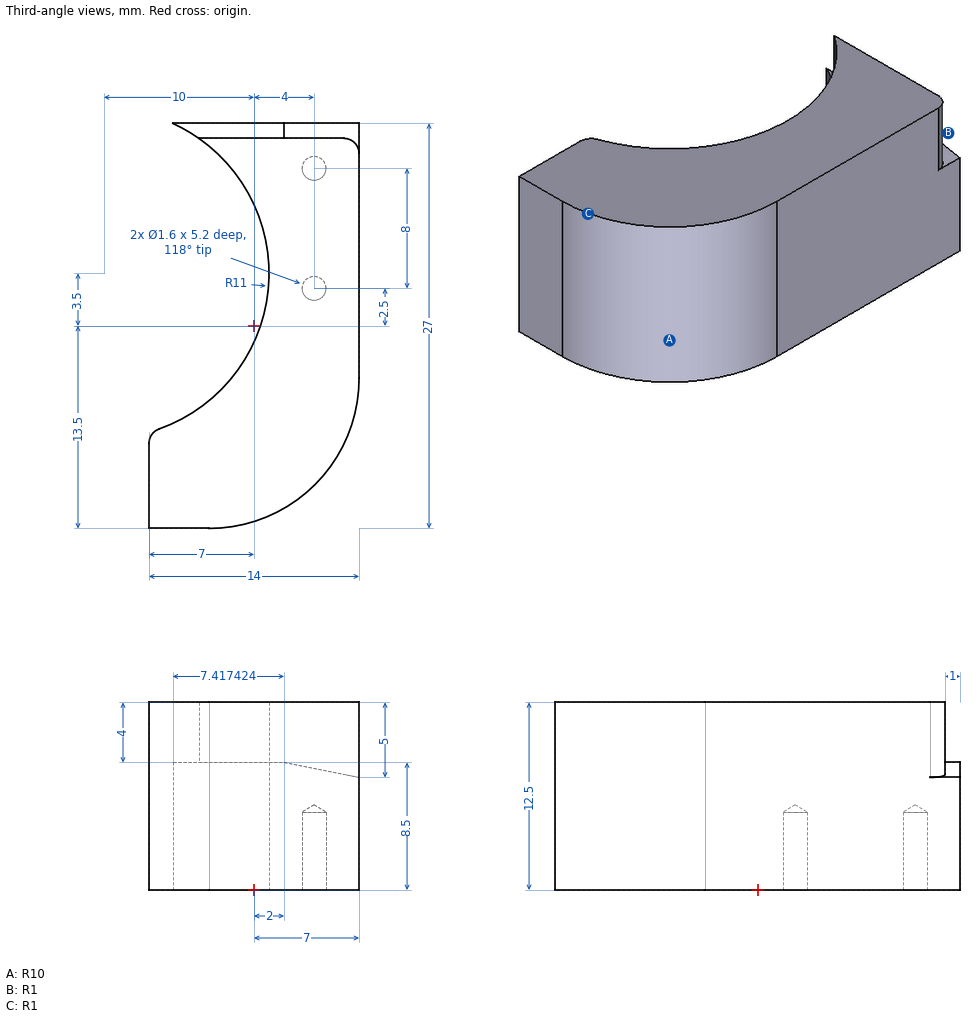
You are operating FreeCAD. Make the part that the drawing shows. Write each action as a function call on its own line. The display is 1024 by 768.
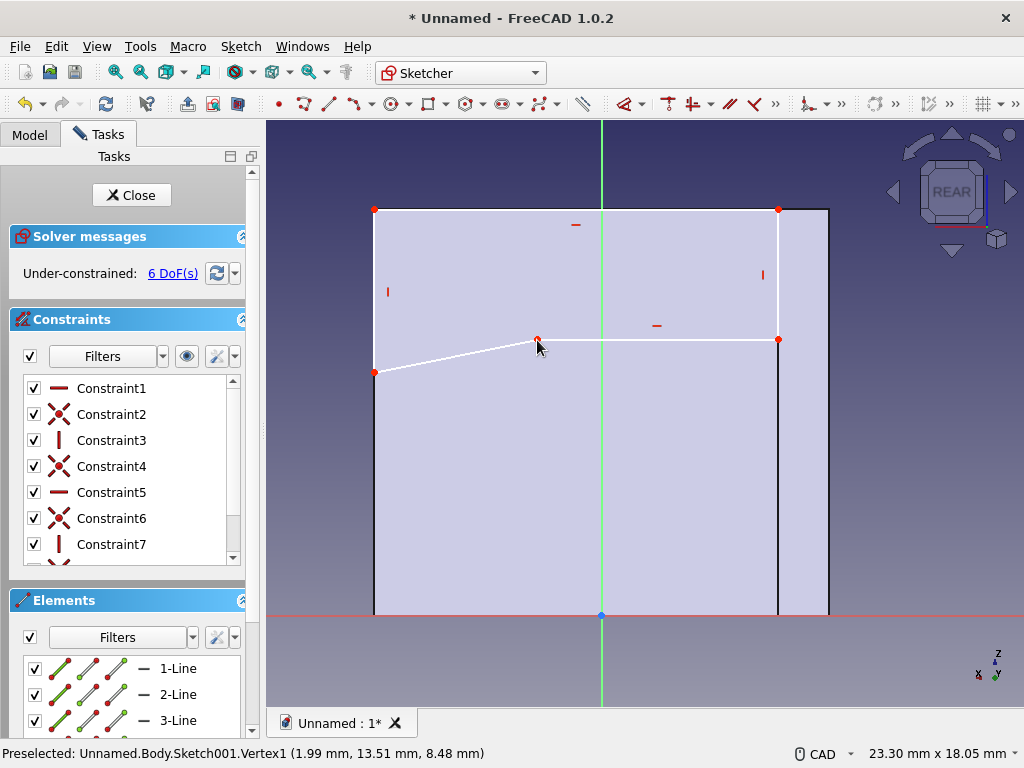
click(624, 104)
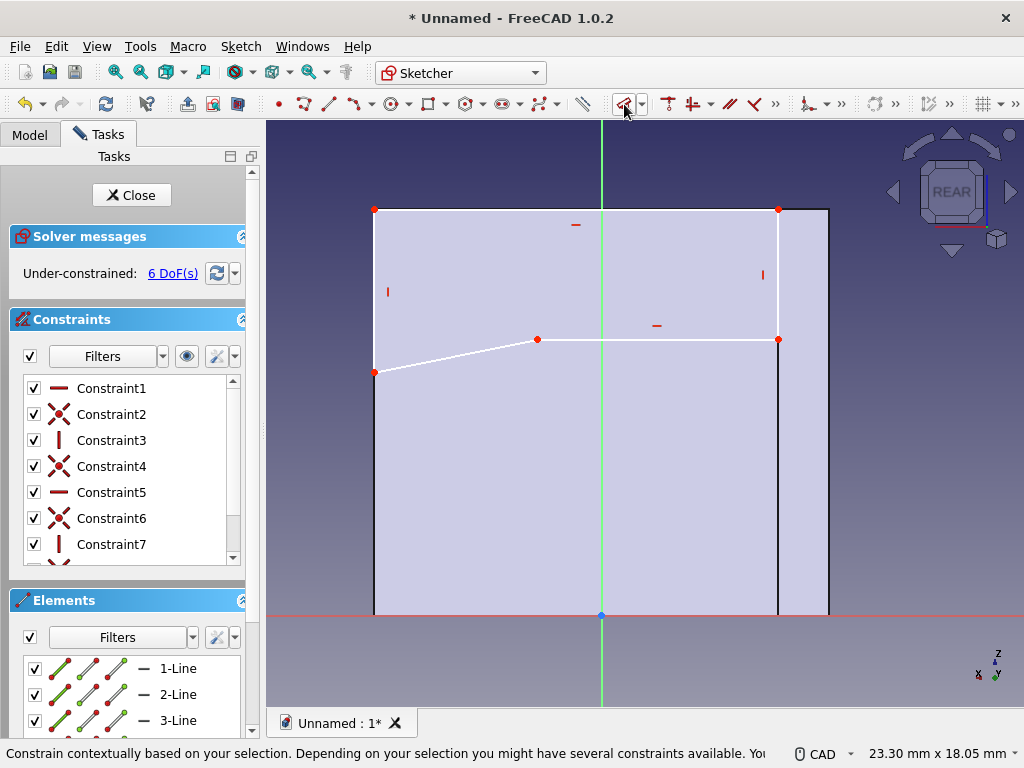
click(778, 301)
click(812, 275)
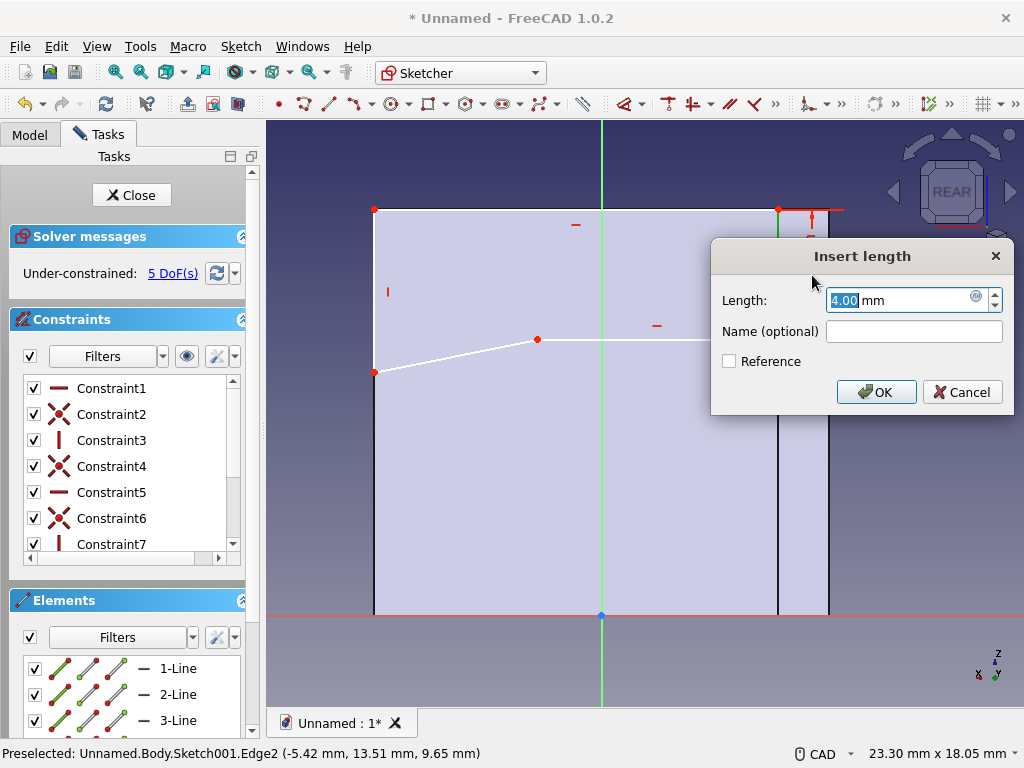
text(4)
key(Return)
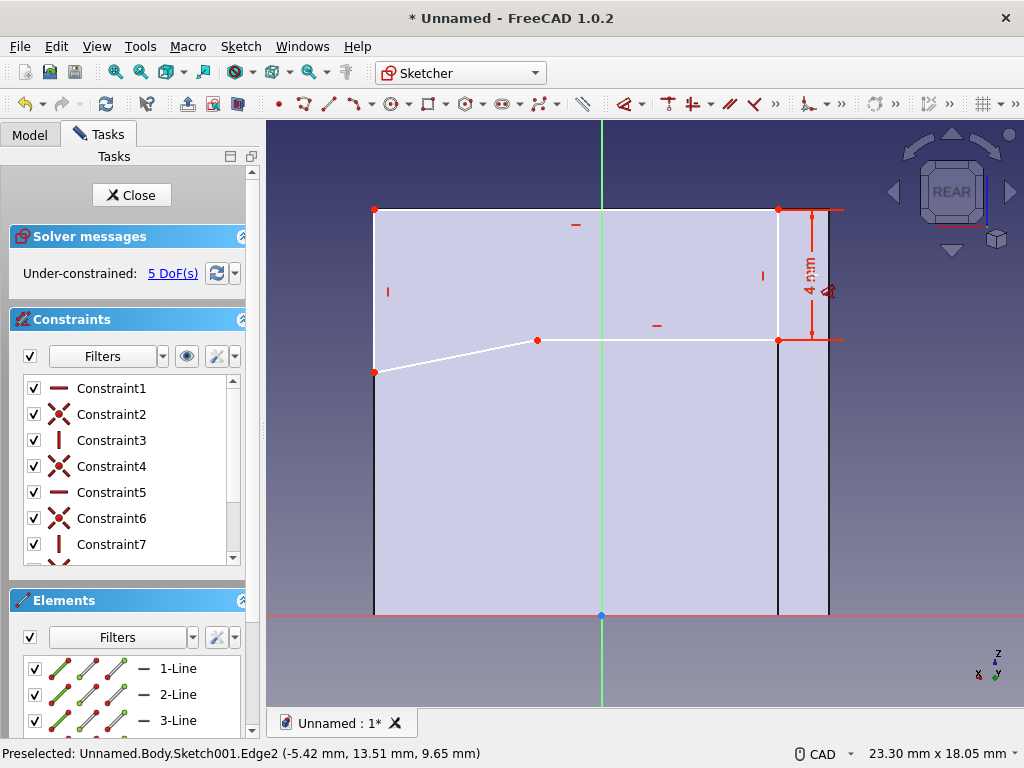
click(374, 259)
click(340, 292)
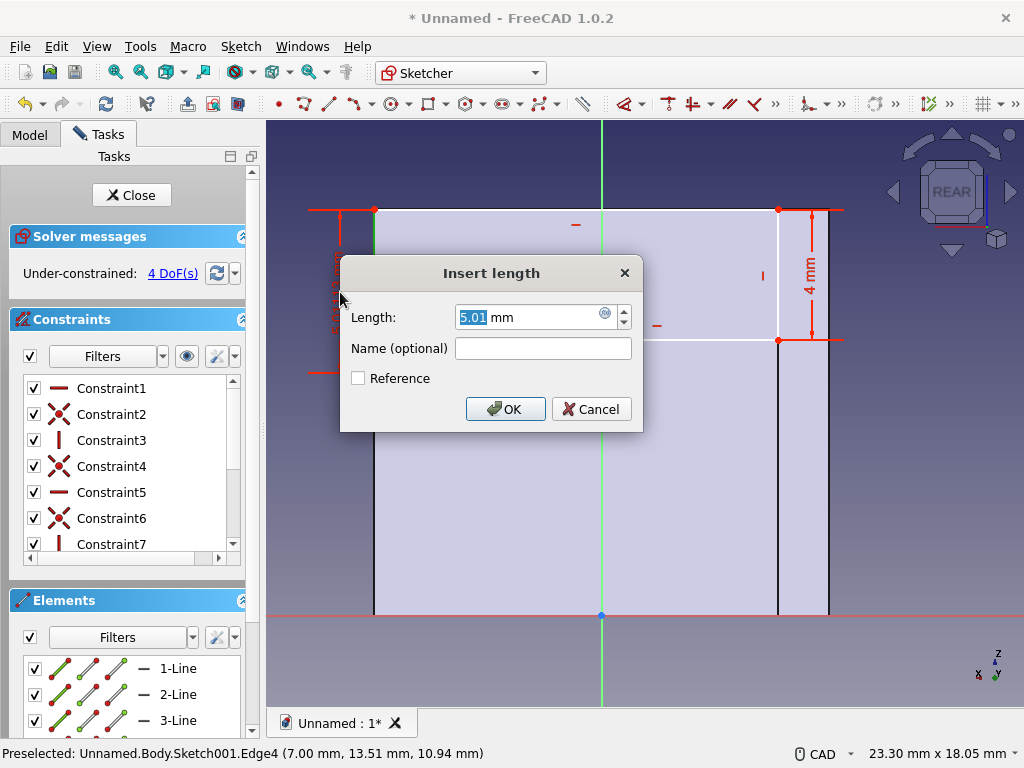
text(5)
key(Return)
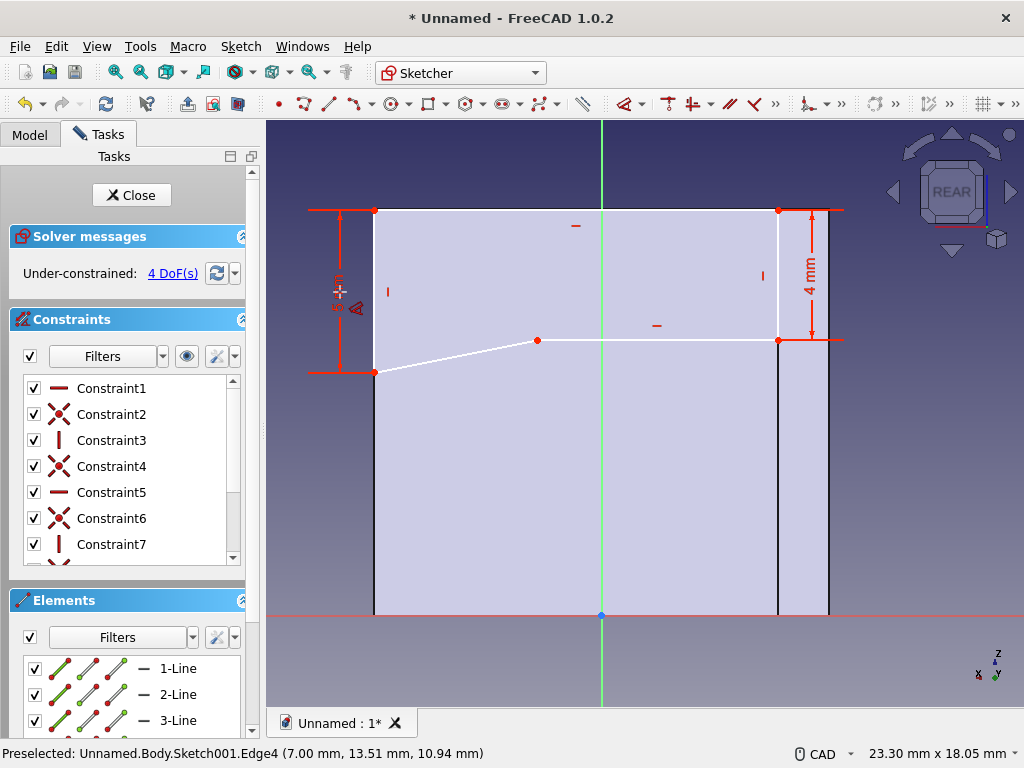
click(537, 340)
click(569, 650)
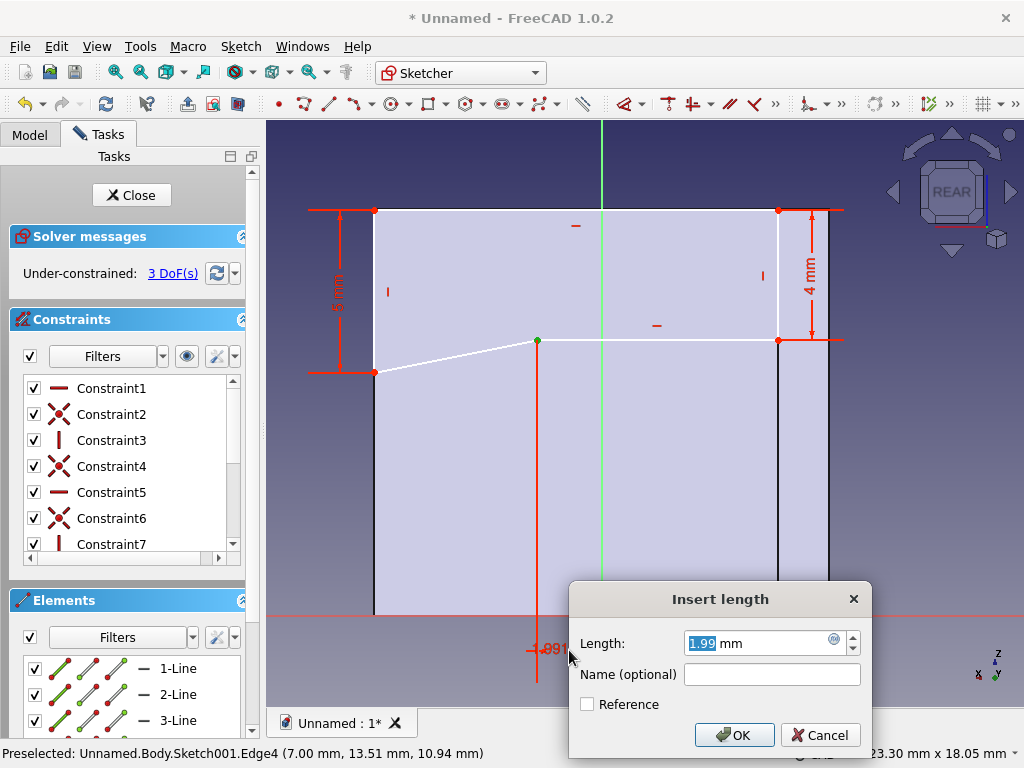
text(2)
key(Return)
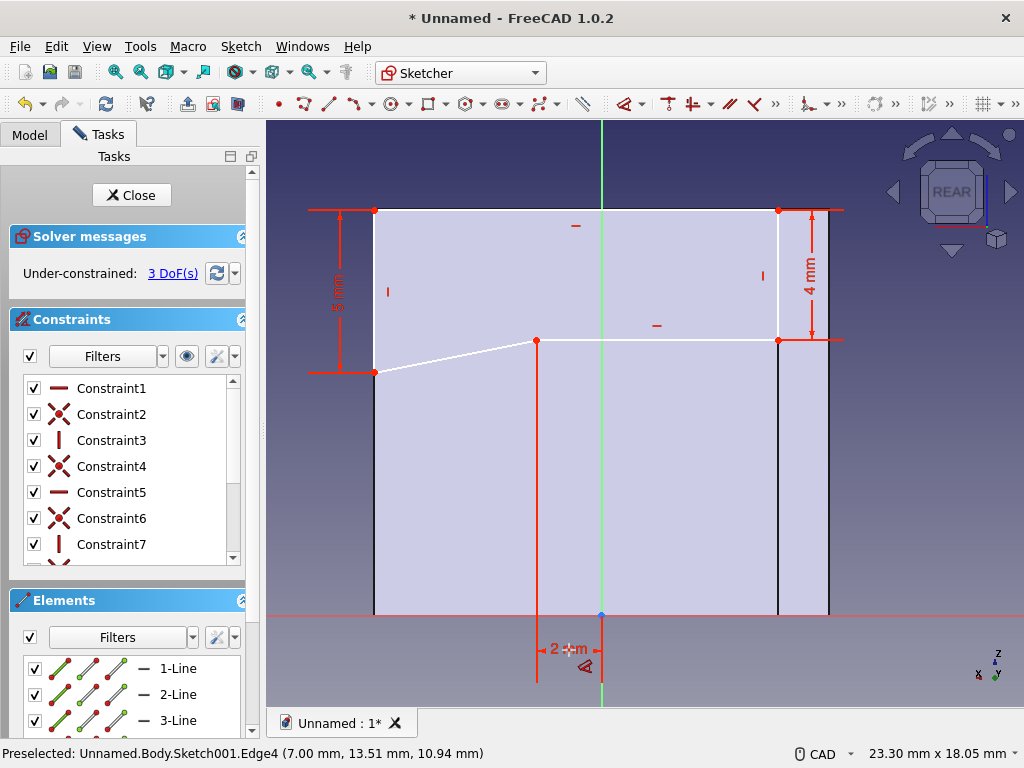
click(374, 210)
click(488, 650)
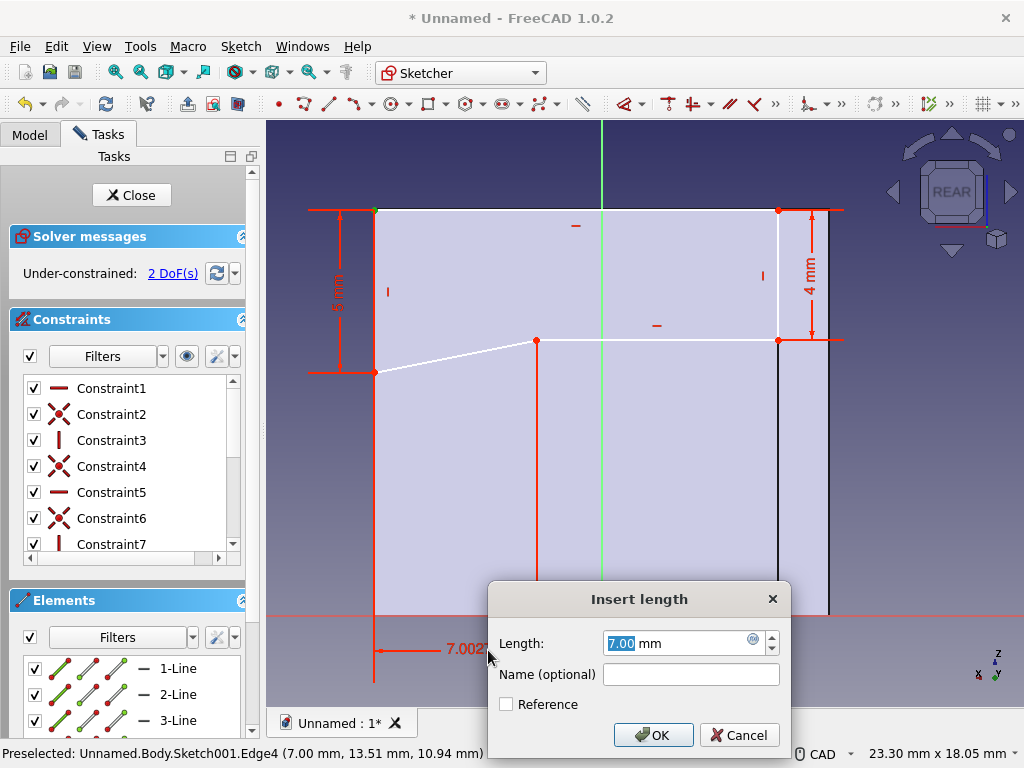
text(7)
key(Return)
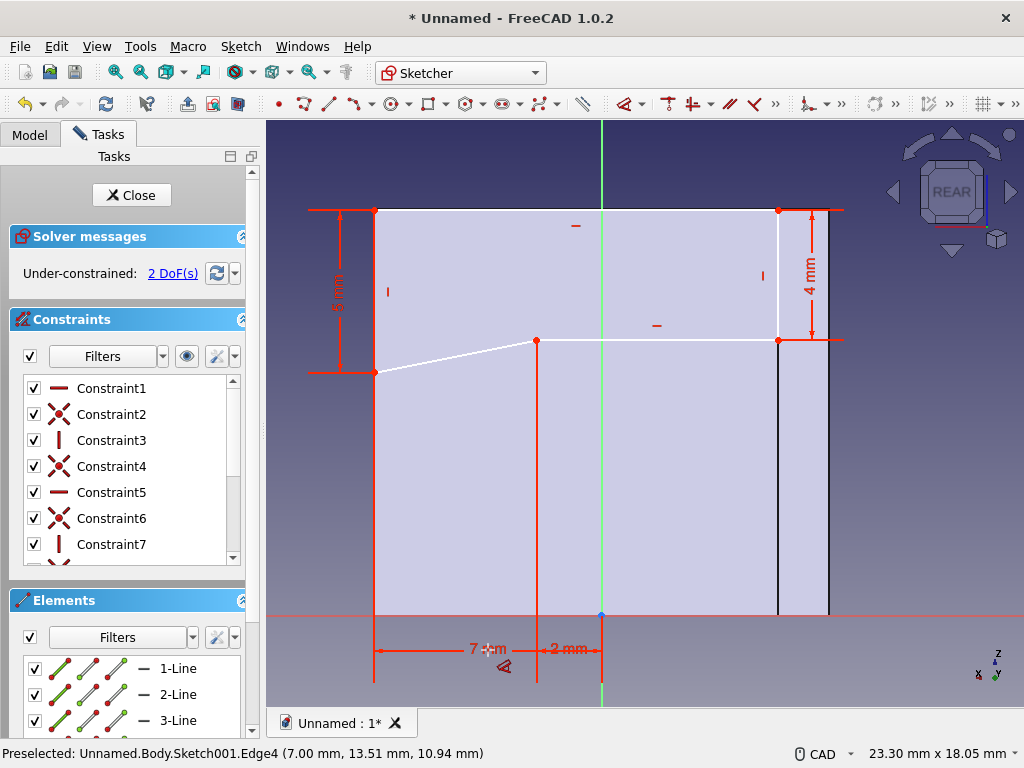
click(537, 340)
click(503, 478)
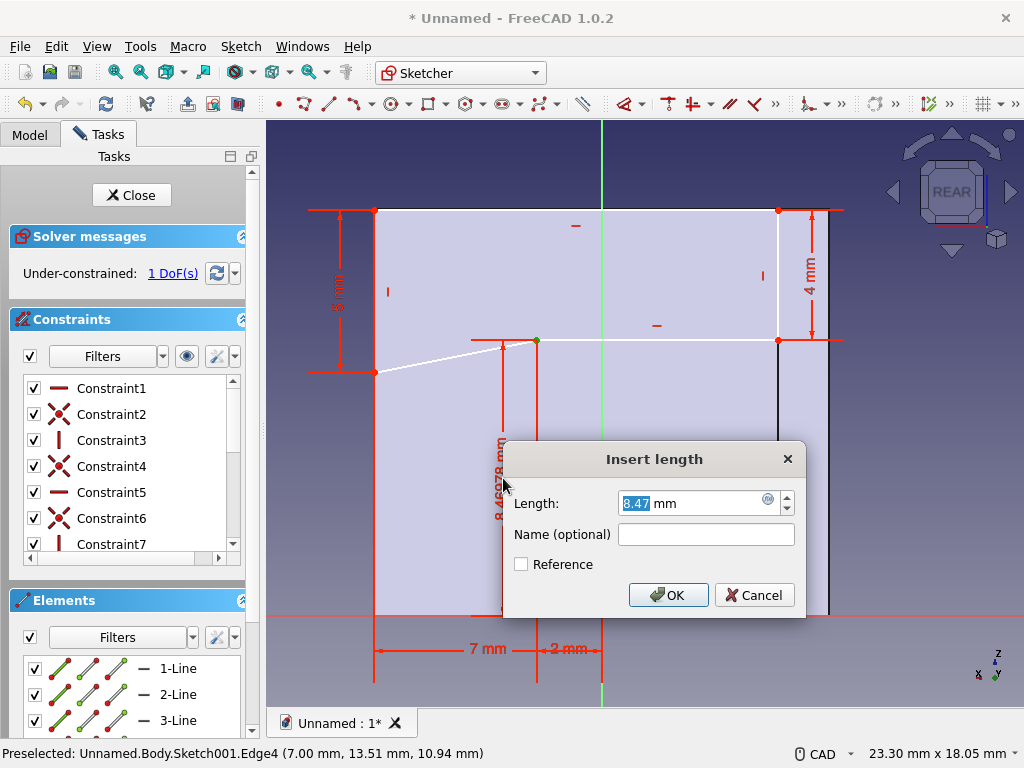
text(8.5)
key(Return)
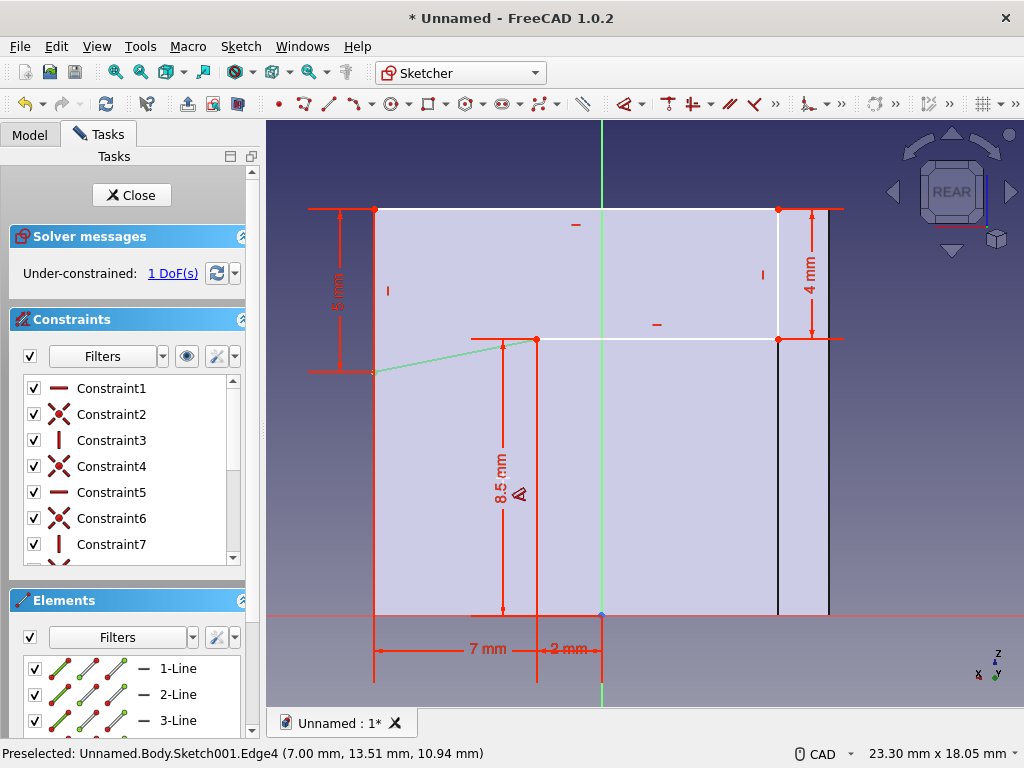
click(706, 339)
click(657, 305)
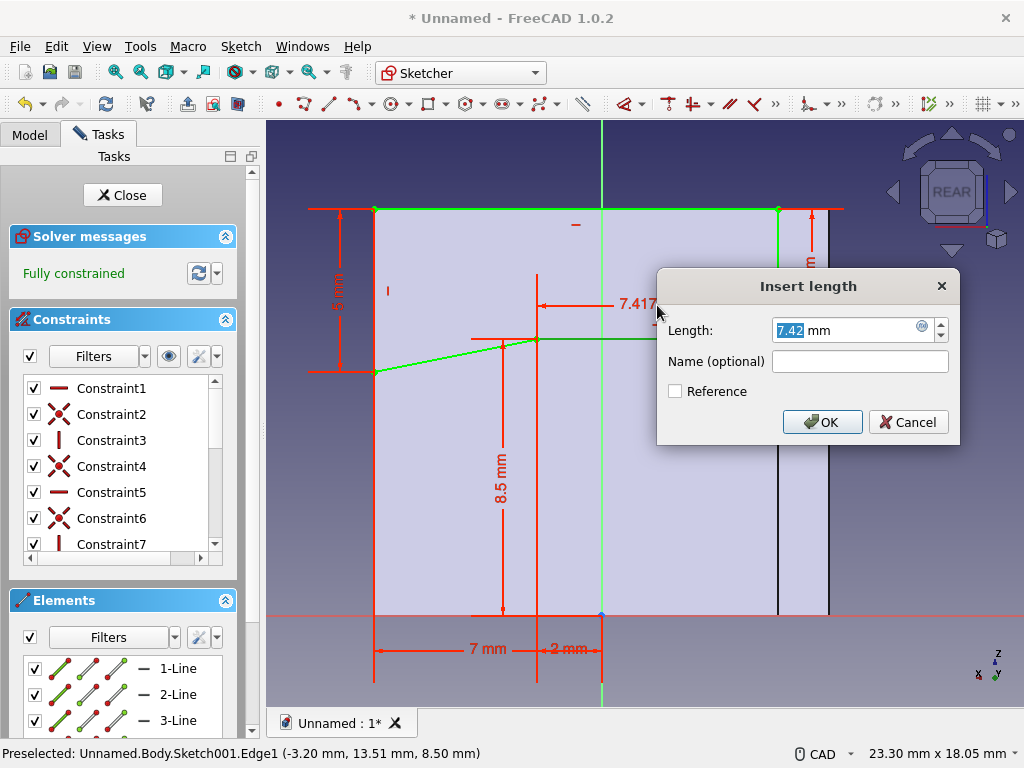
text(7.417424)
key(Return)
key(Escape)